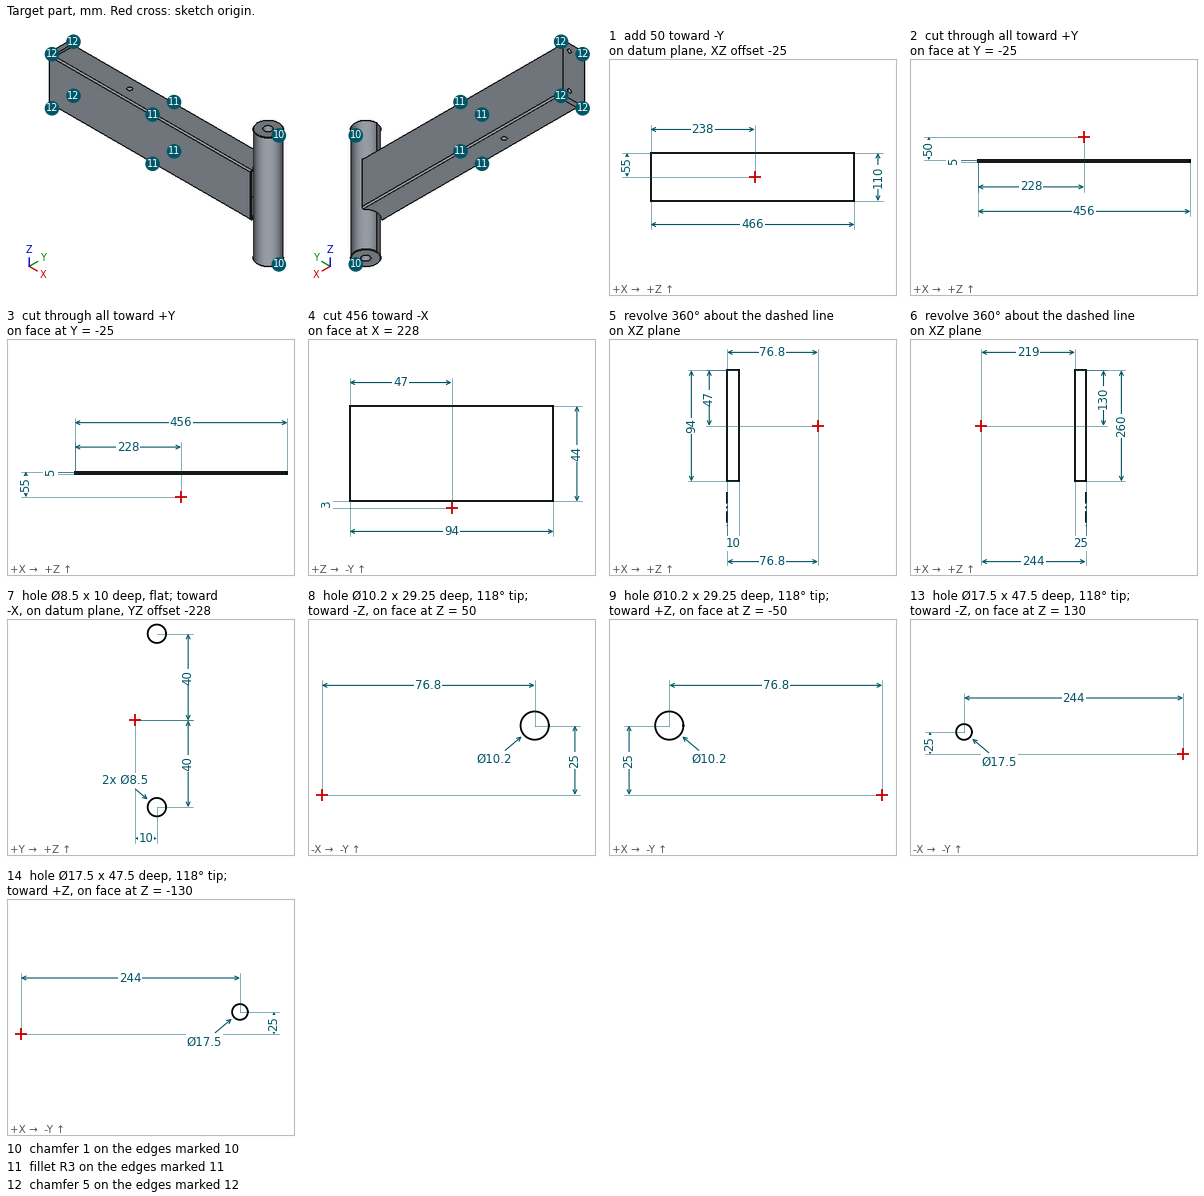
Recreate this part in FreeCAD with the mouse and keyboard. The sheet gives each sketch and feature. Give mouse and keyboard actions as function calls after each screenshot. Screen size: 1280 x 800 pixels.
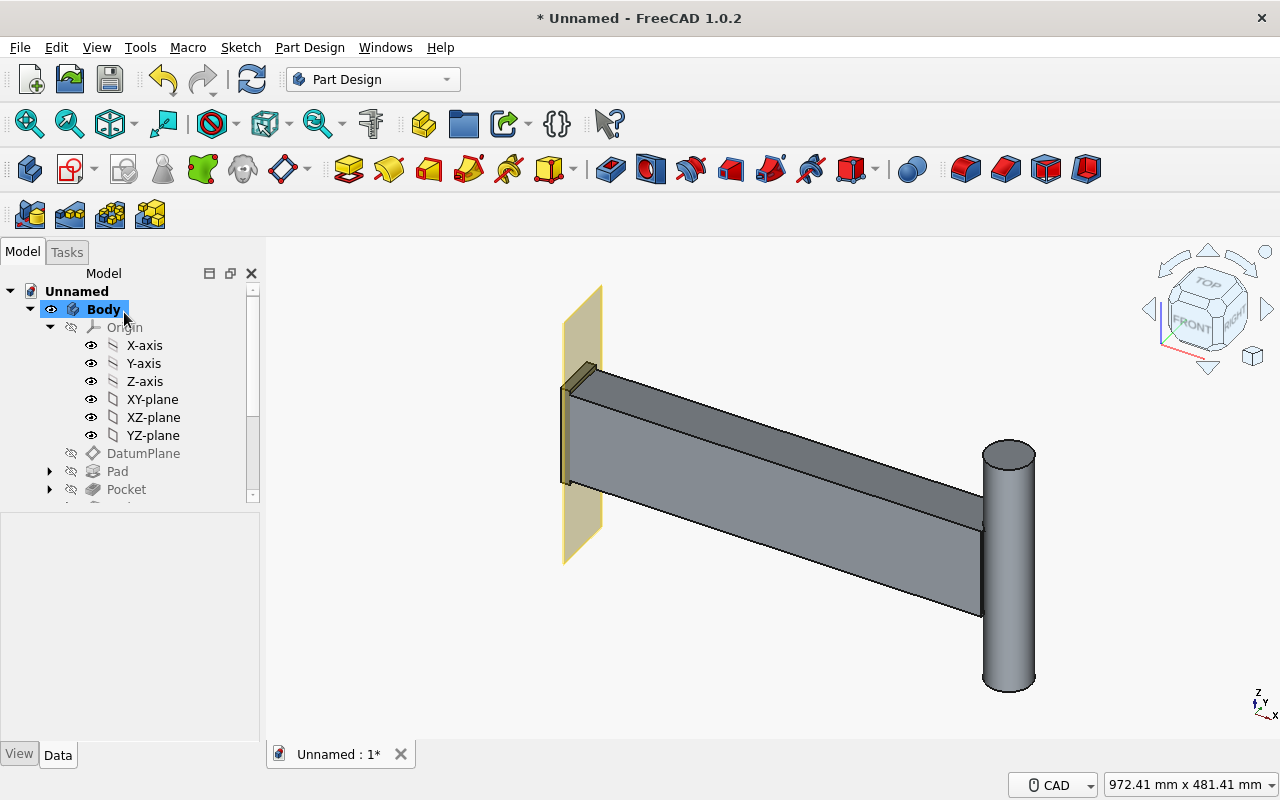
scroll(100, 395, down, 3)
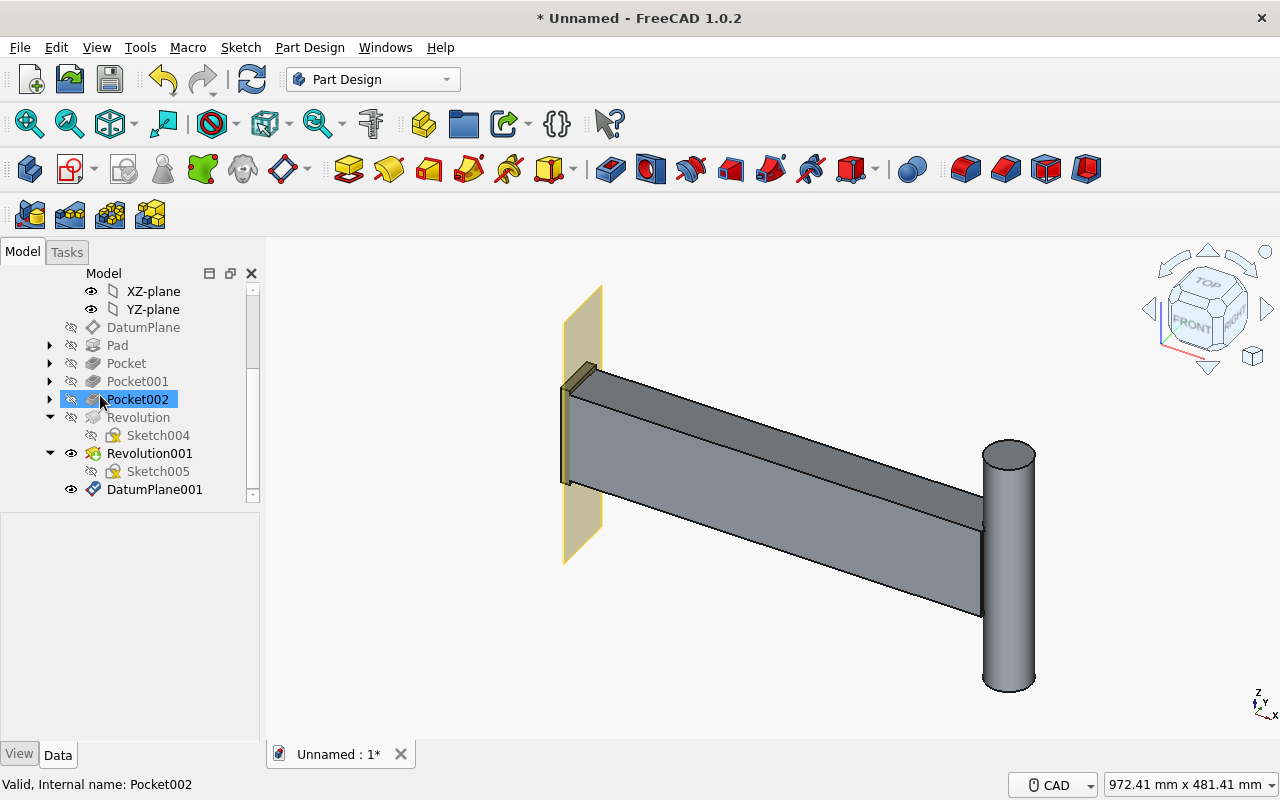
click(116, 489)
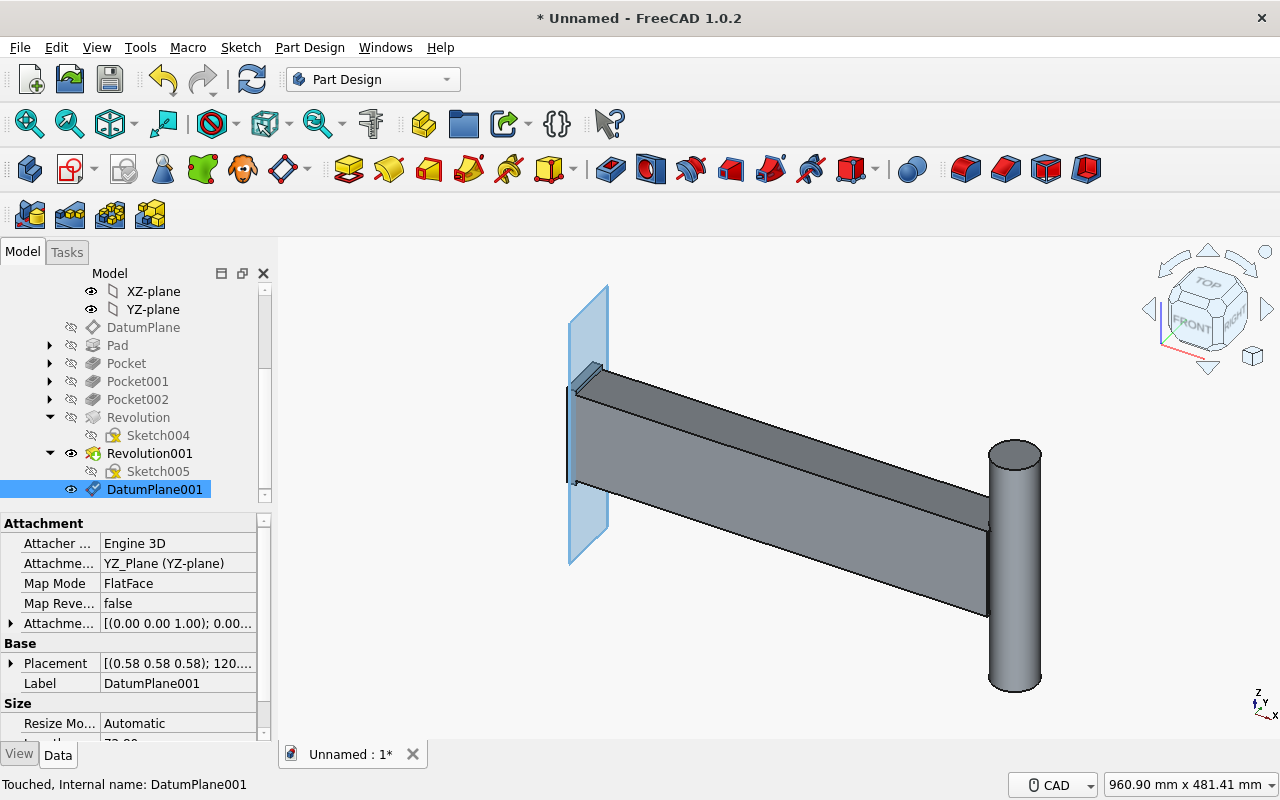
click(70, 170)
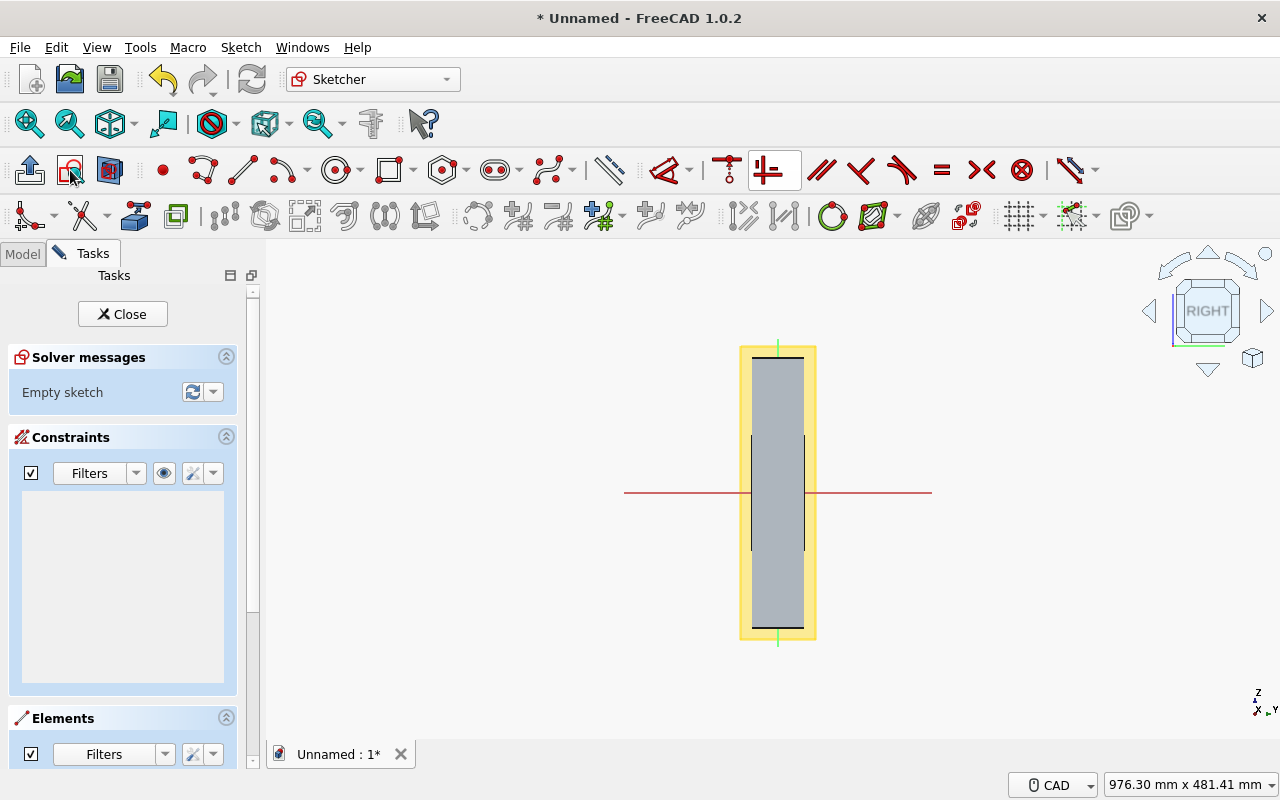
click(110, 170)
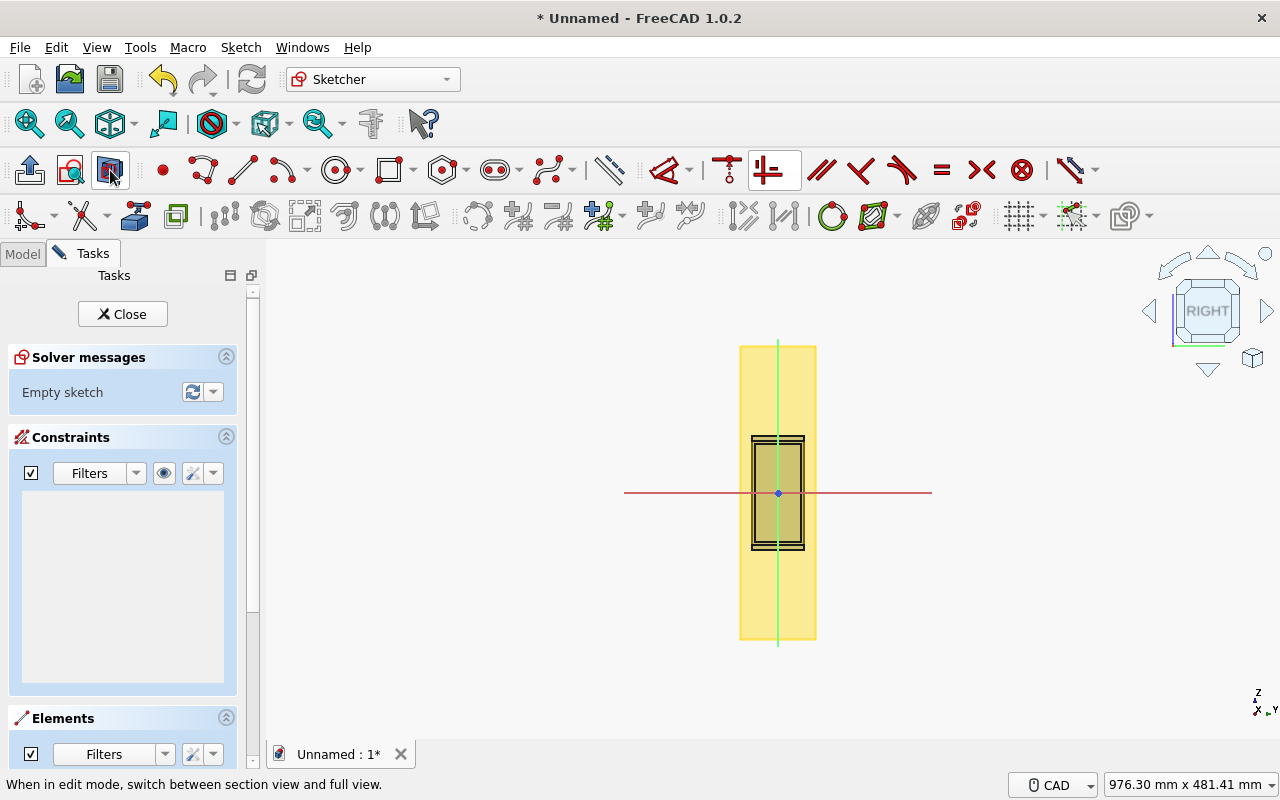
scroll(820, 495, up, 6)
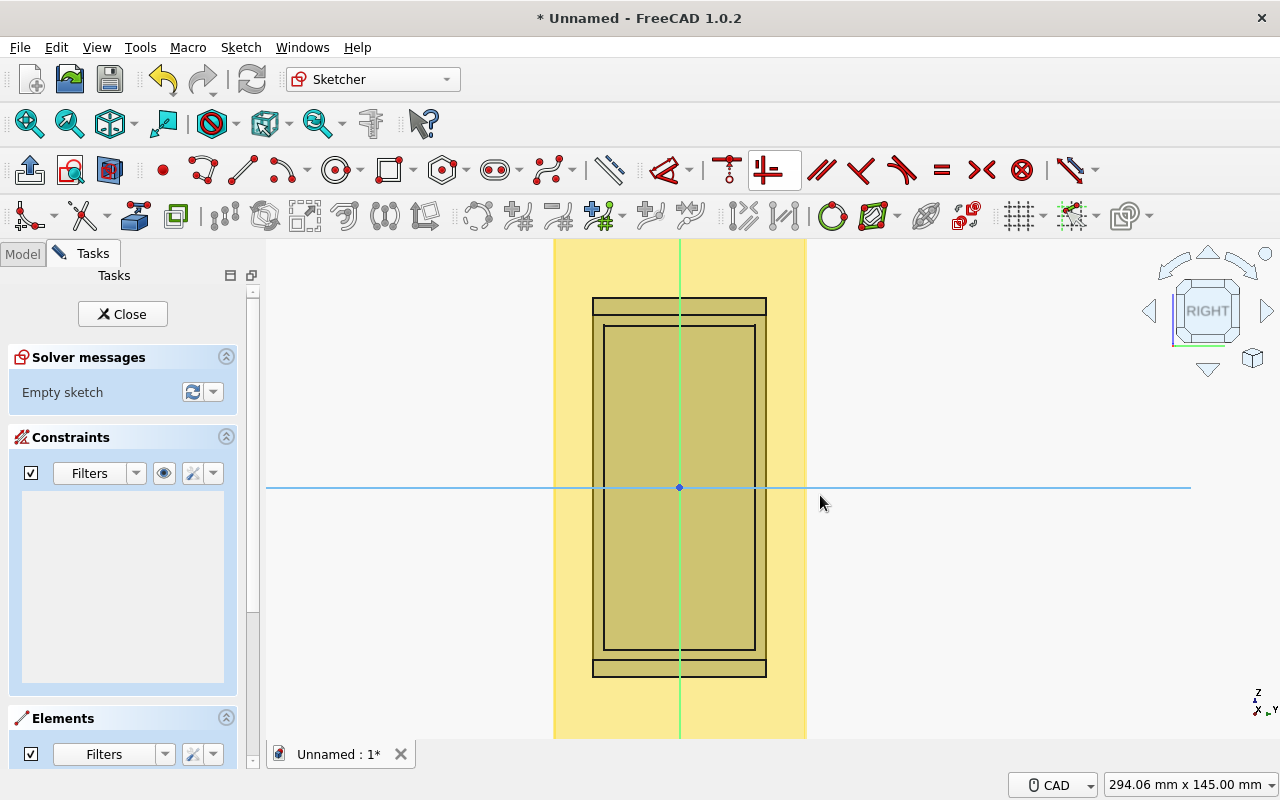
click(336, 170)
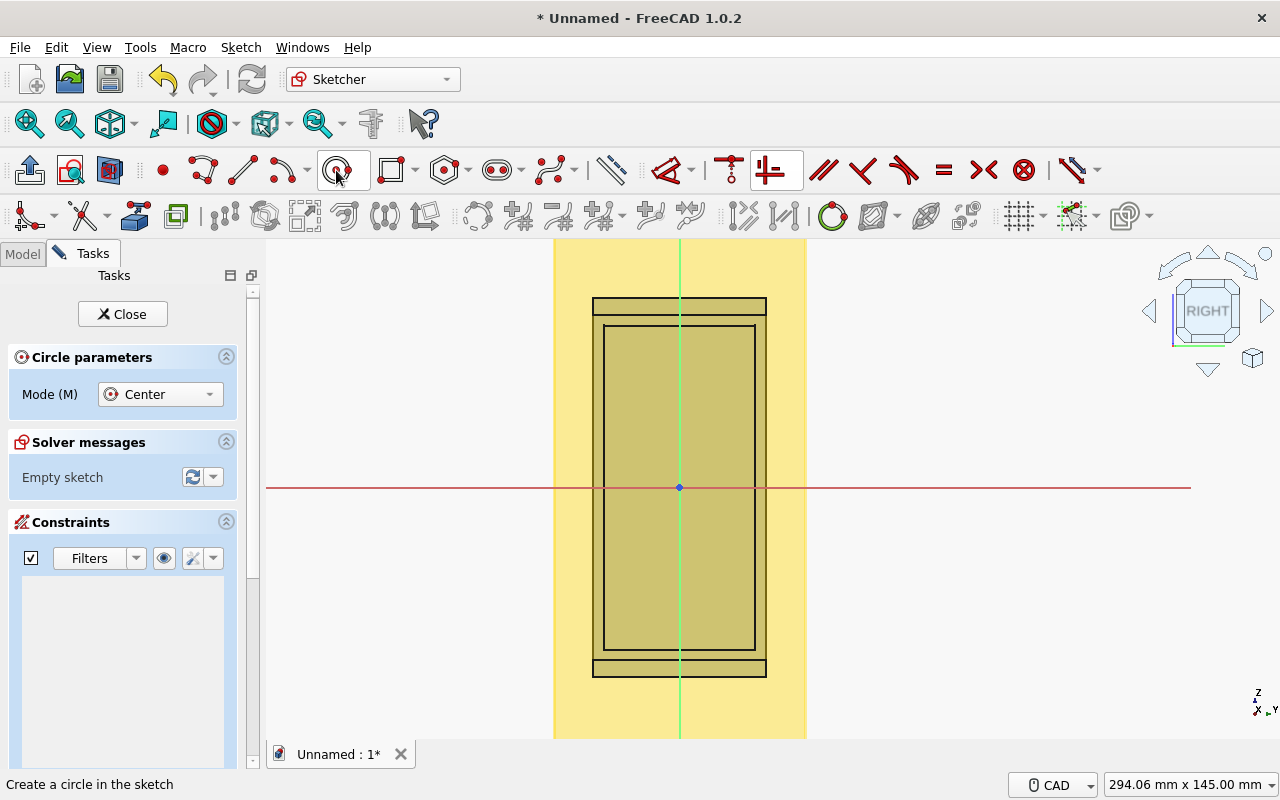
scroll(714, 626, up, 3)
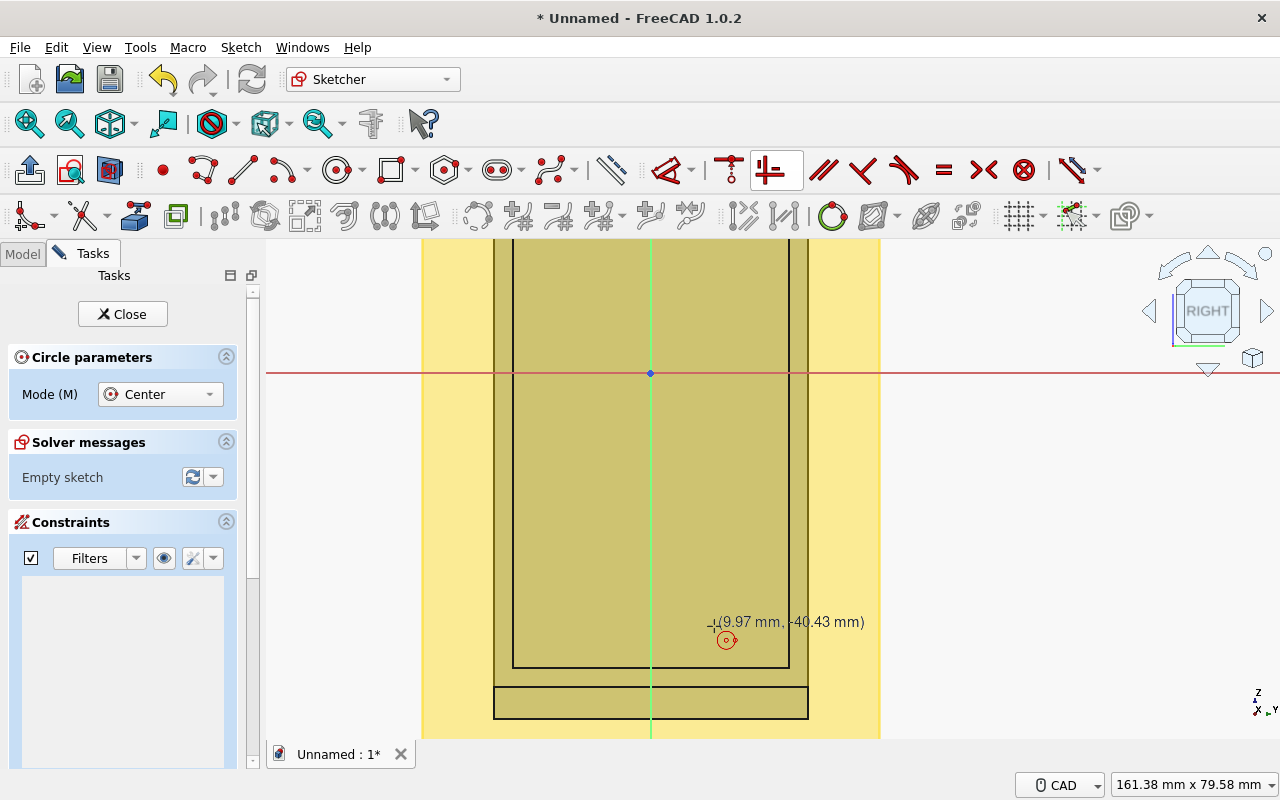
click(714, 624)
move(733, 606)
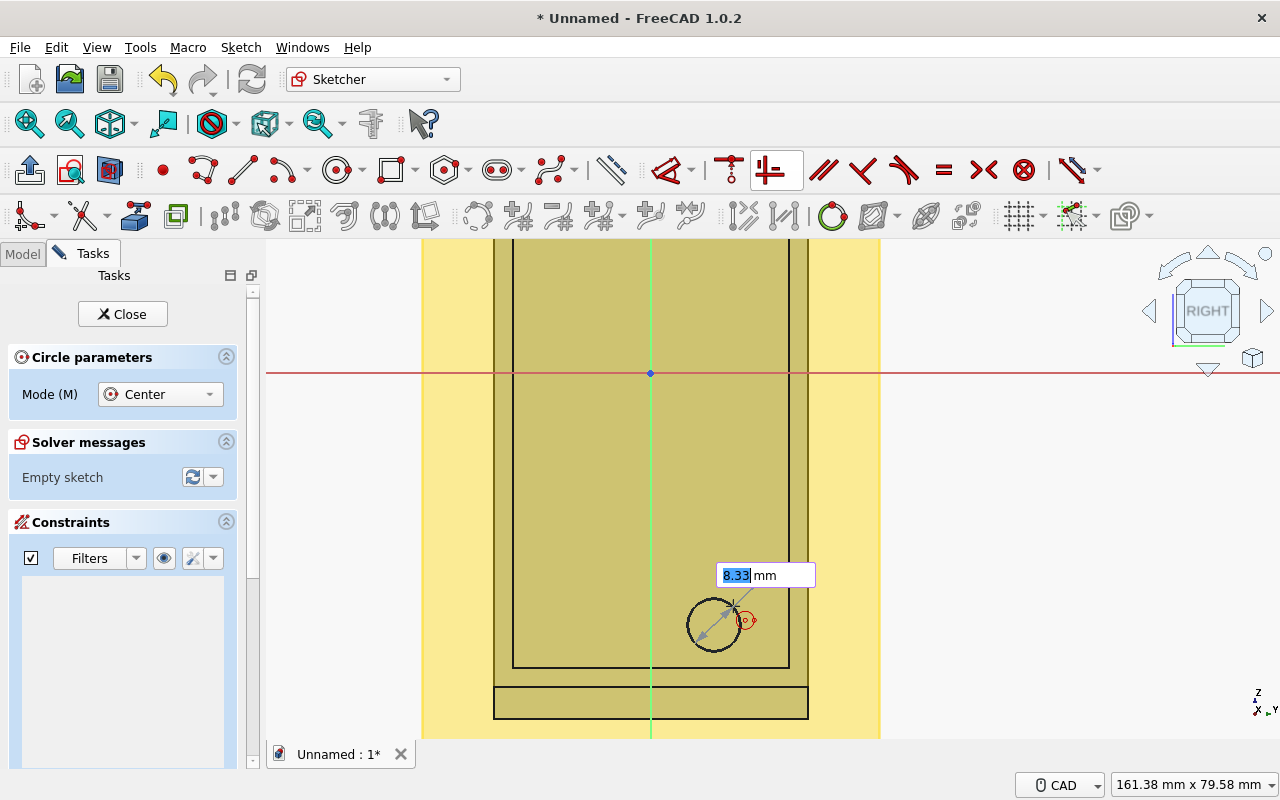
text(8.5)
key(Return)